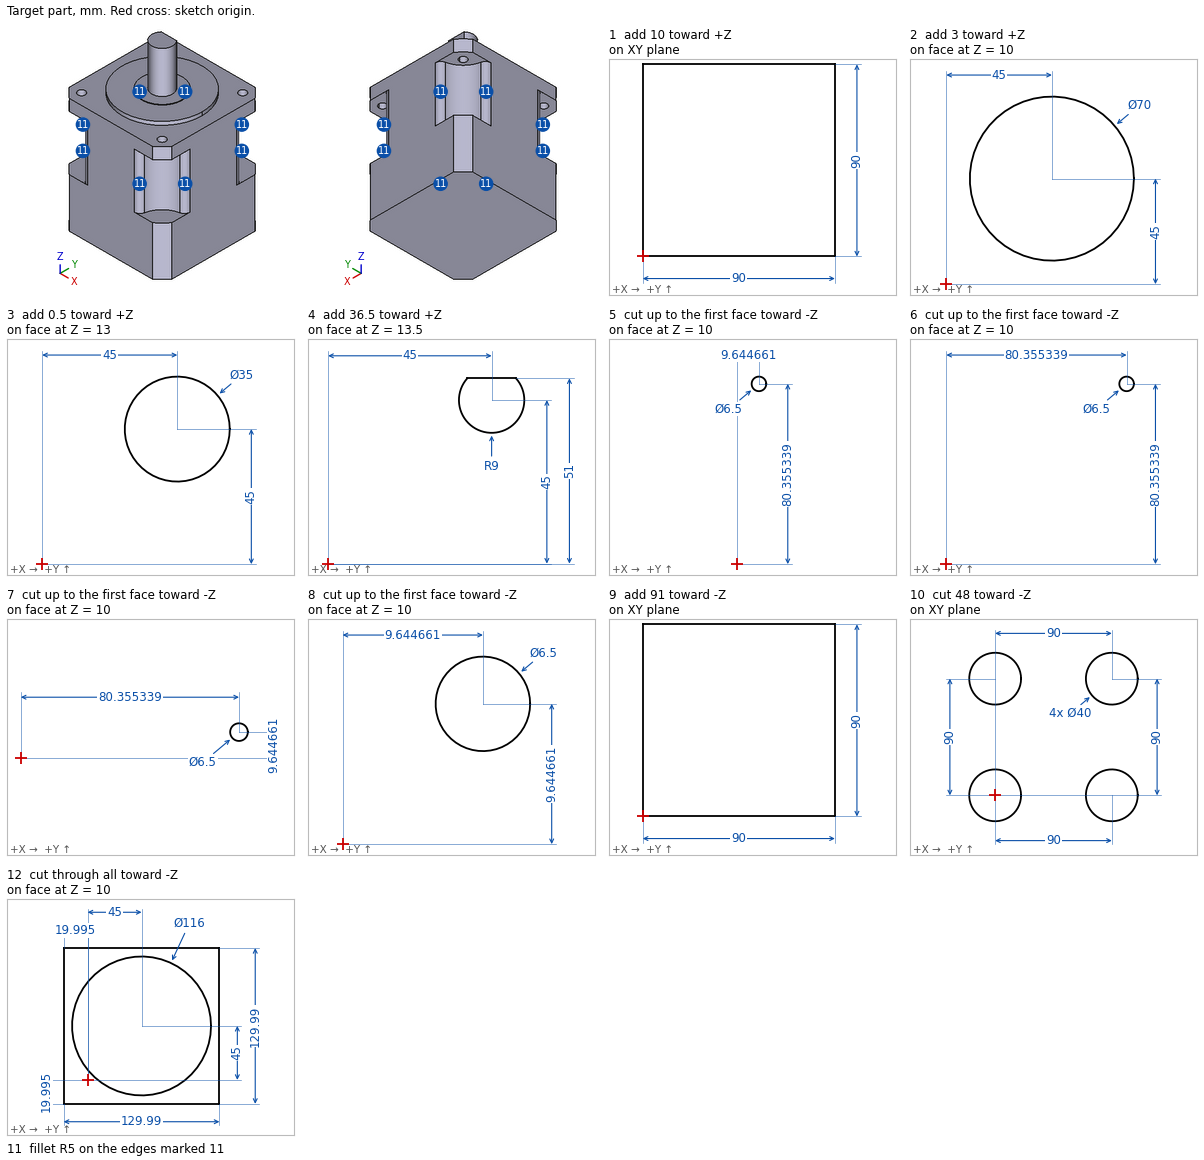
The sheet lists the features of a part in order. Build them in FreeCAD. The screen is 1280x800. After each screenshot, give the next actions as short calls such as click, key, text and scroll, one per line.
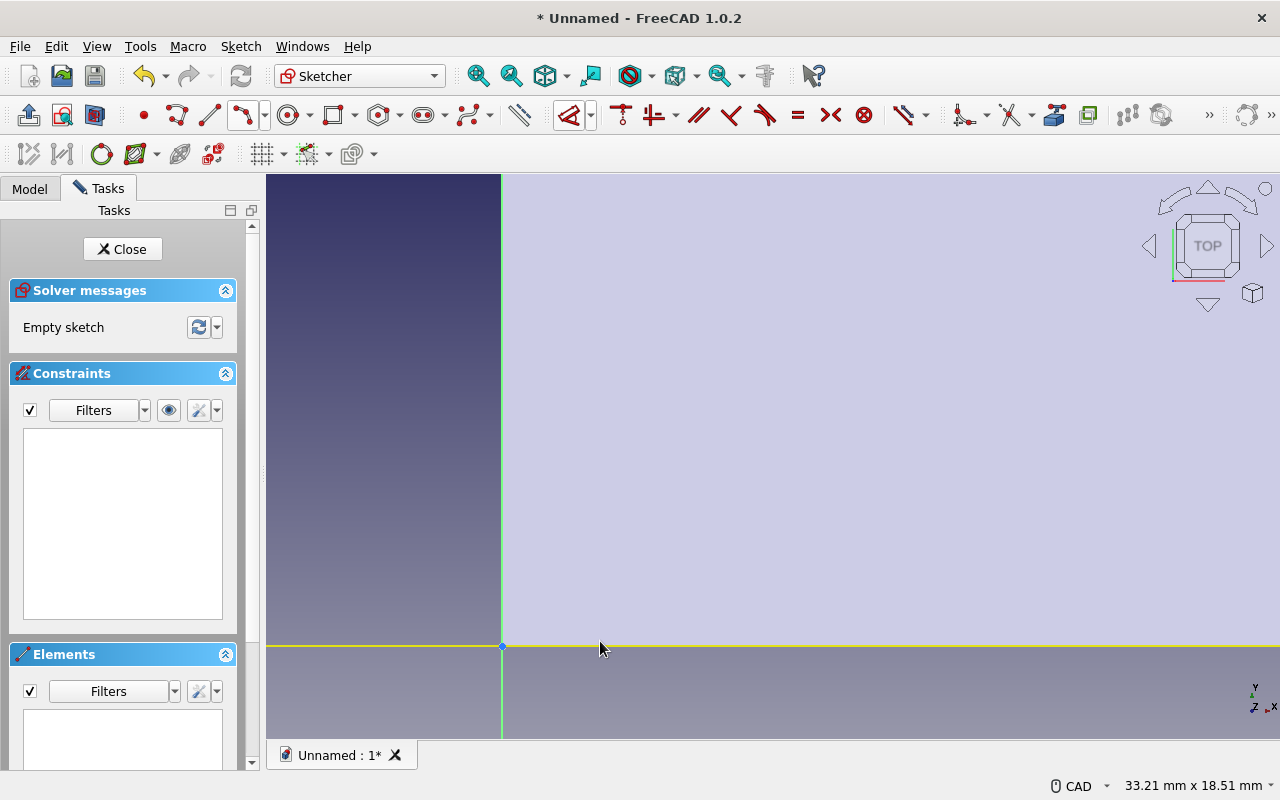
key(g)
key(c)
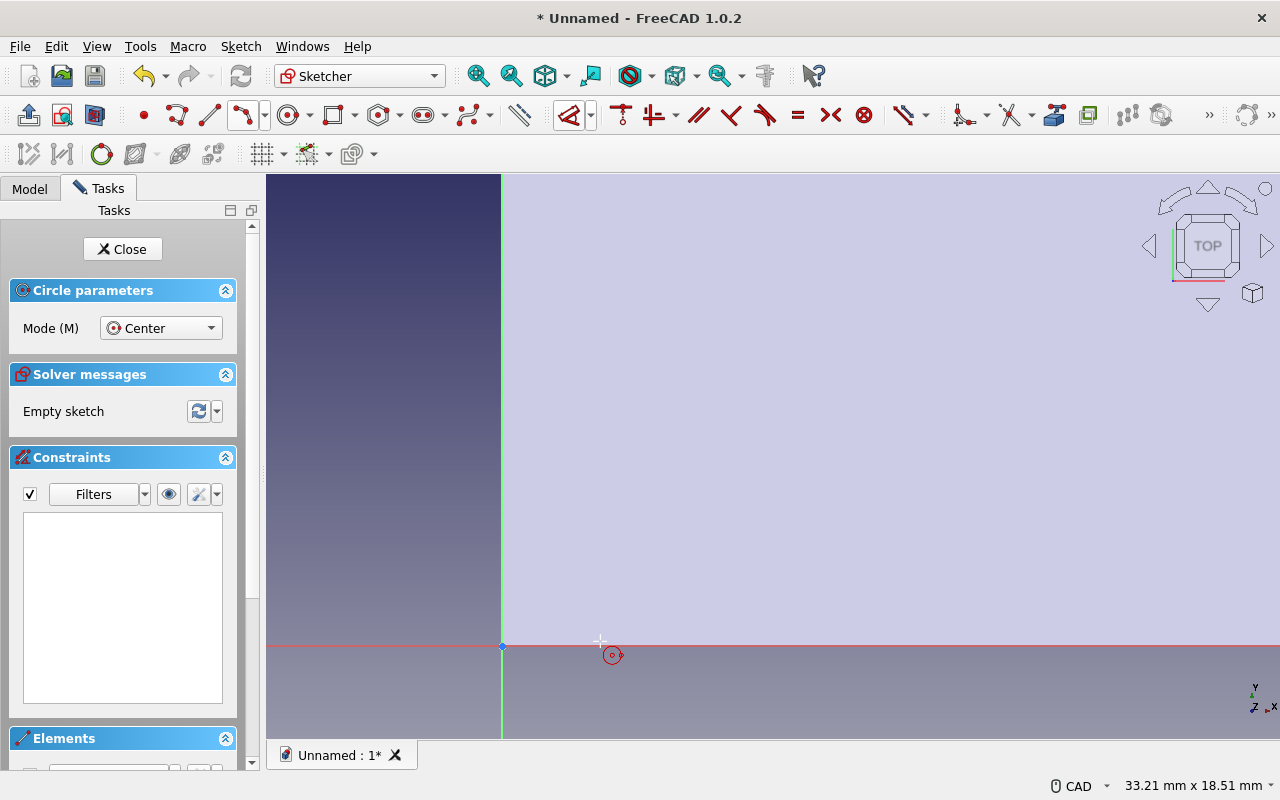
click(797, 352)
move(867, 282)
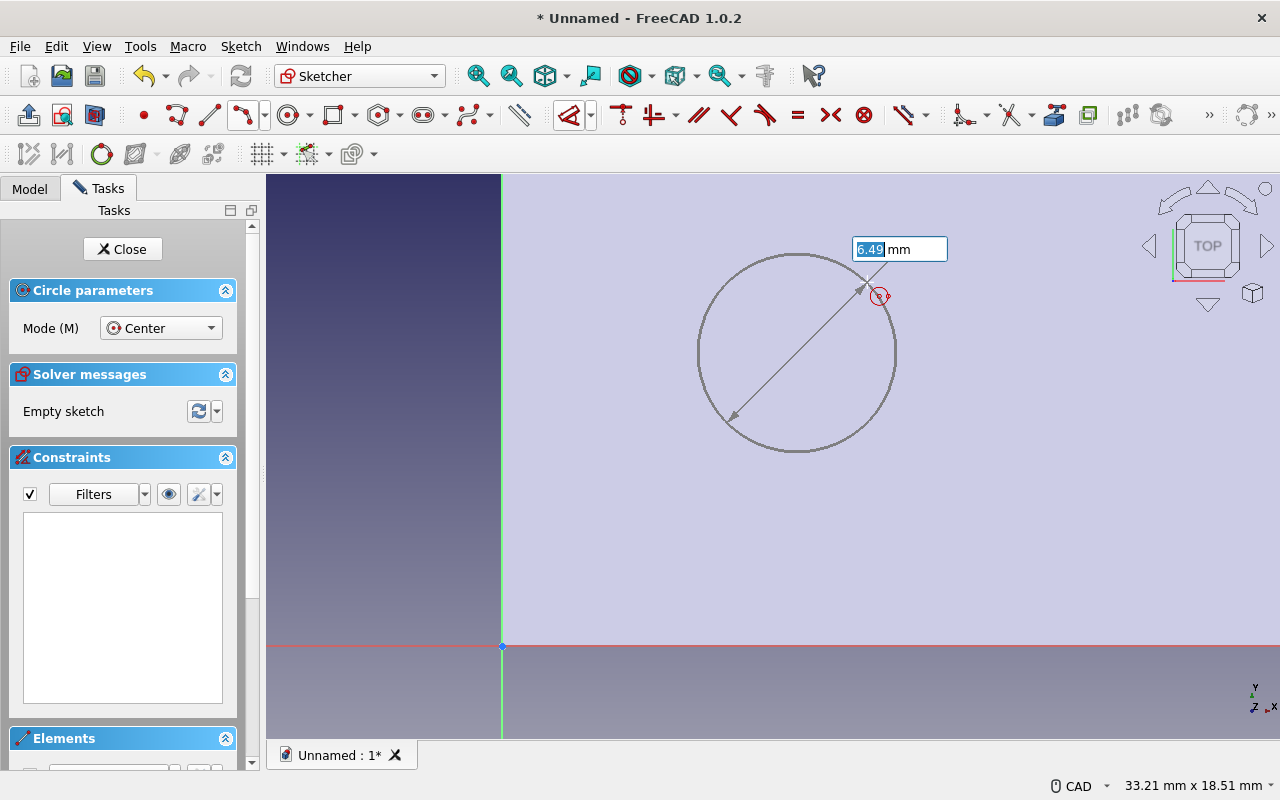
text(6.5)
key(Return)
key(Escape)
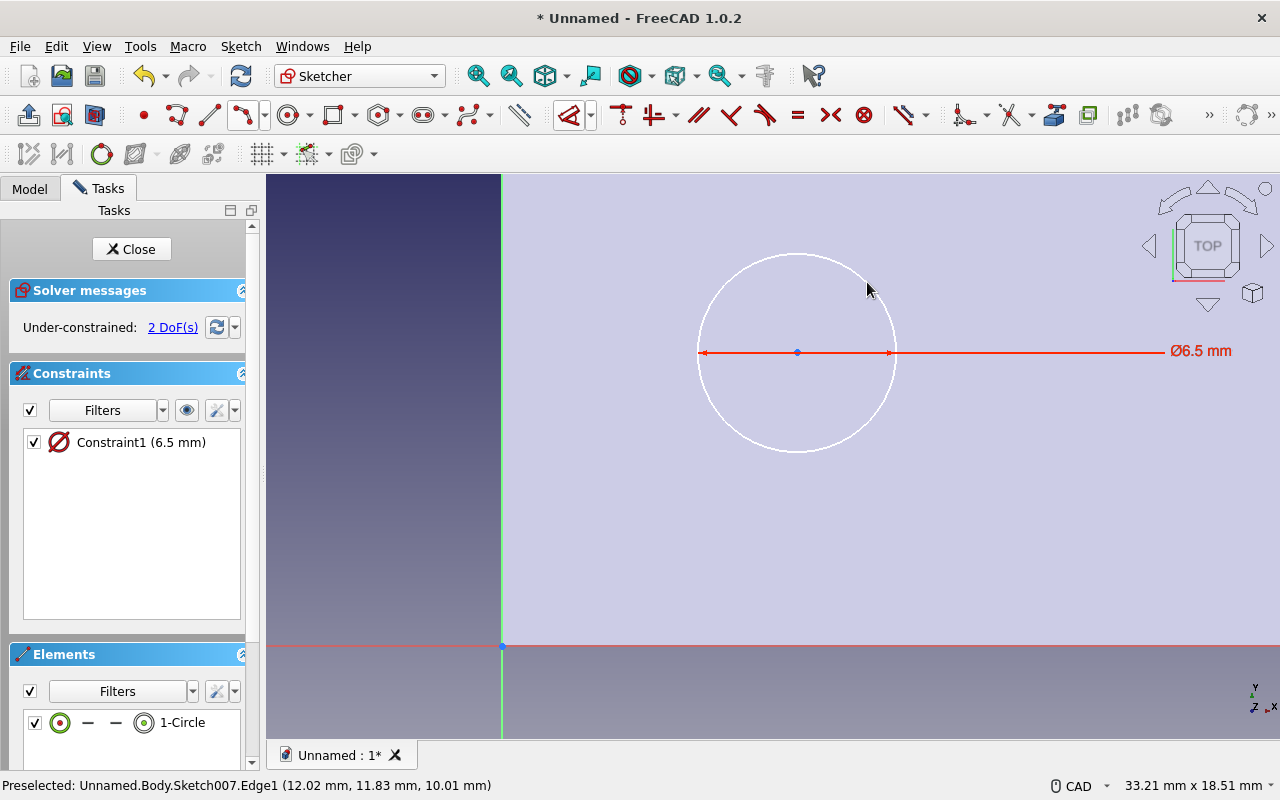
click(797, 353)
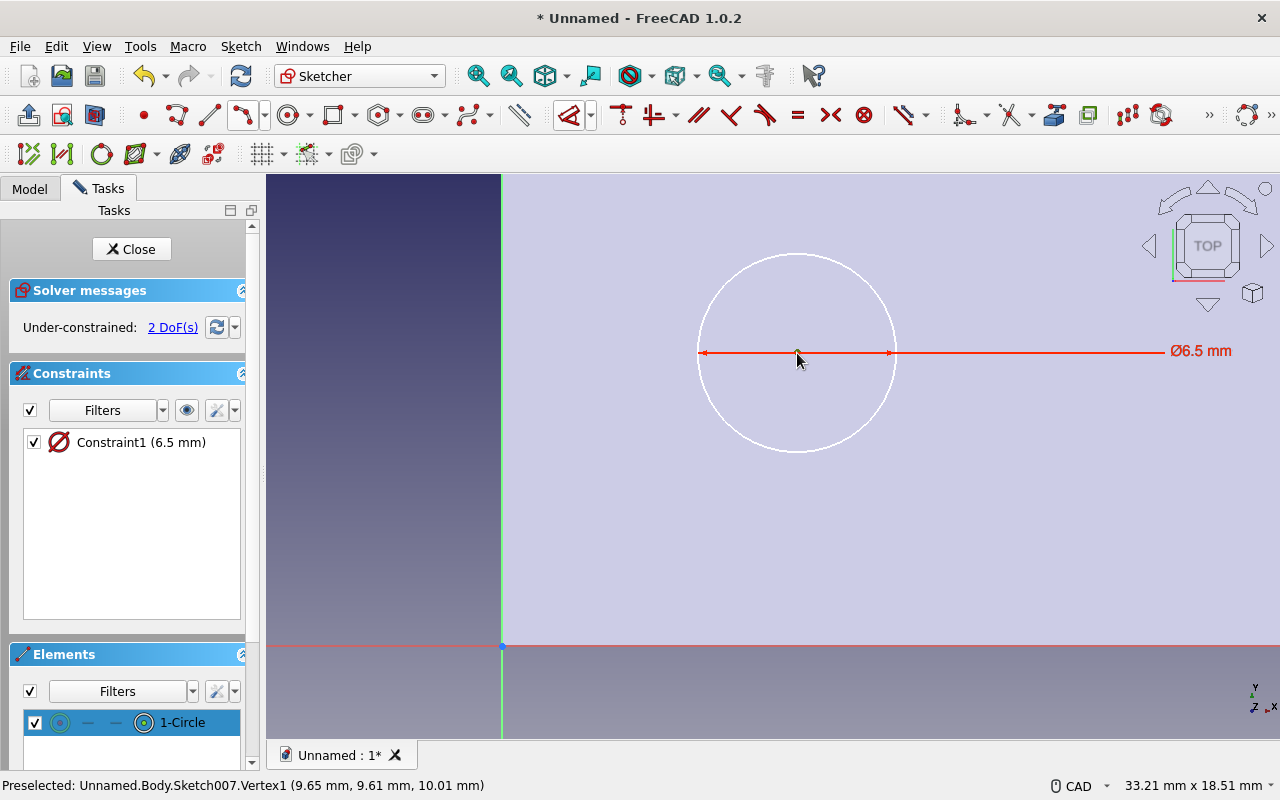
key(l)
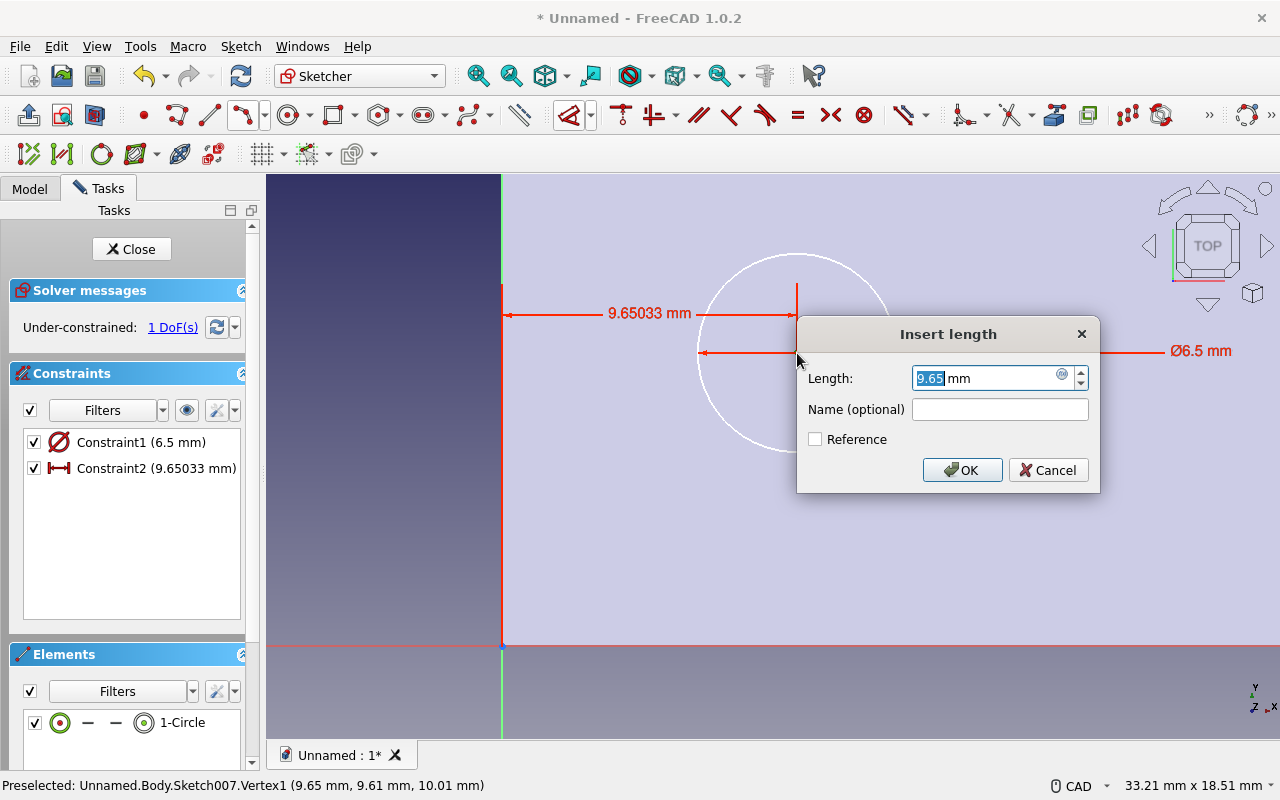
text(9.644661)
key(Return)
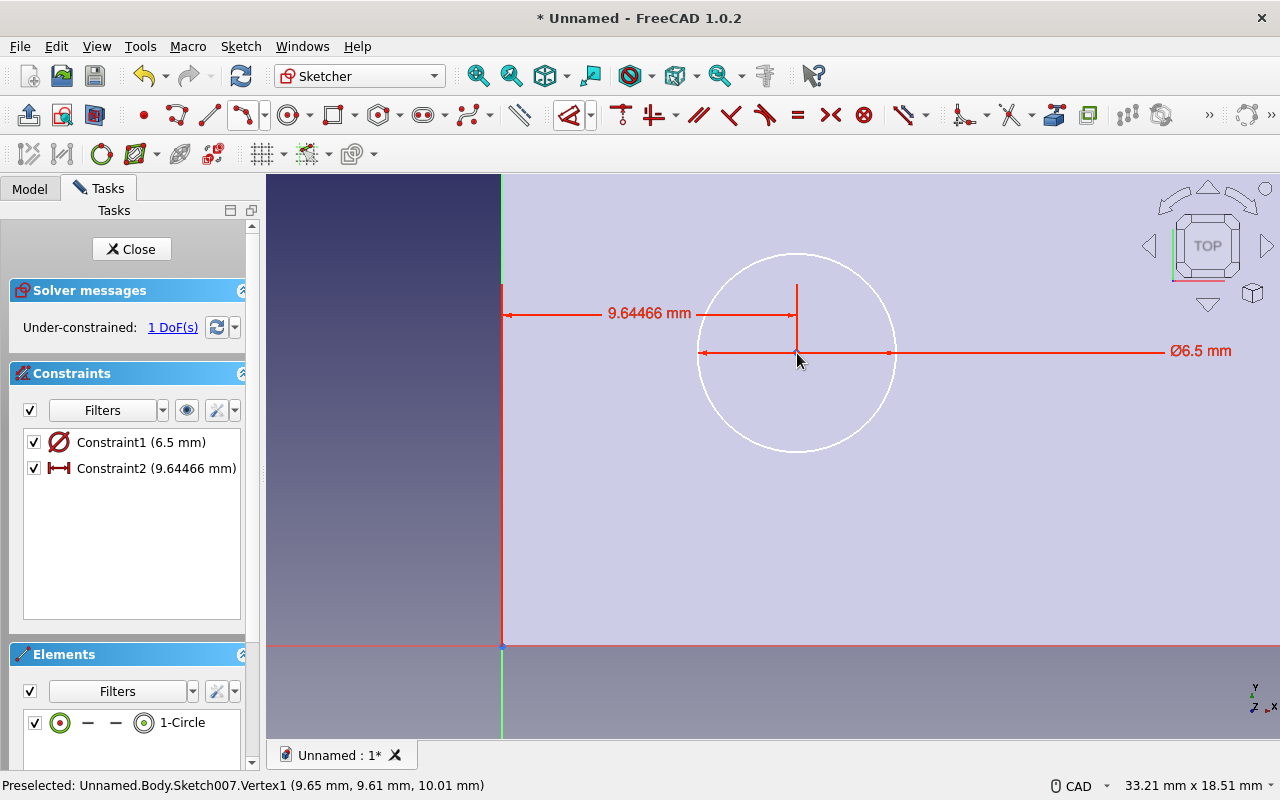
click(797, 353)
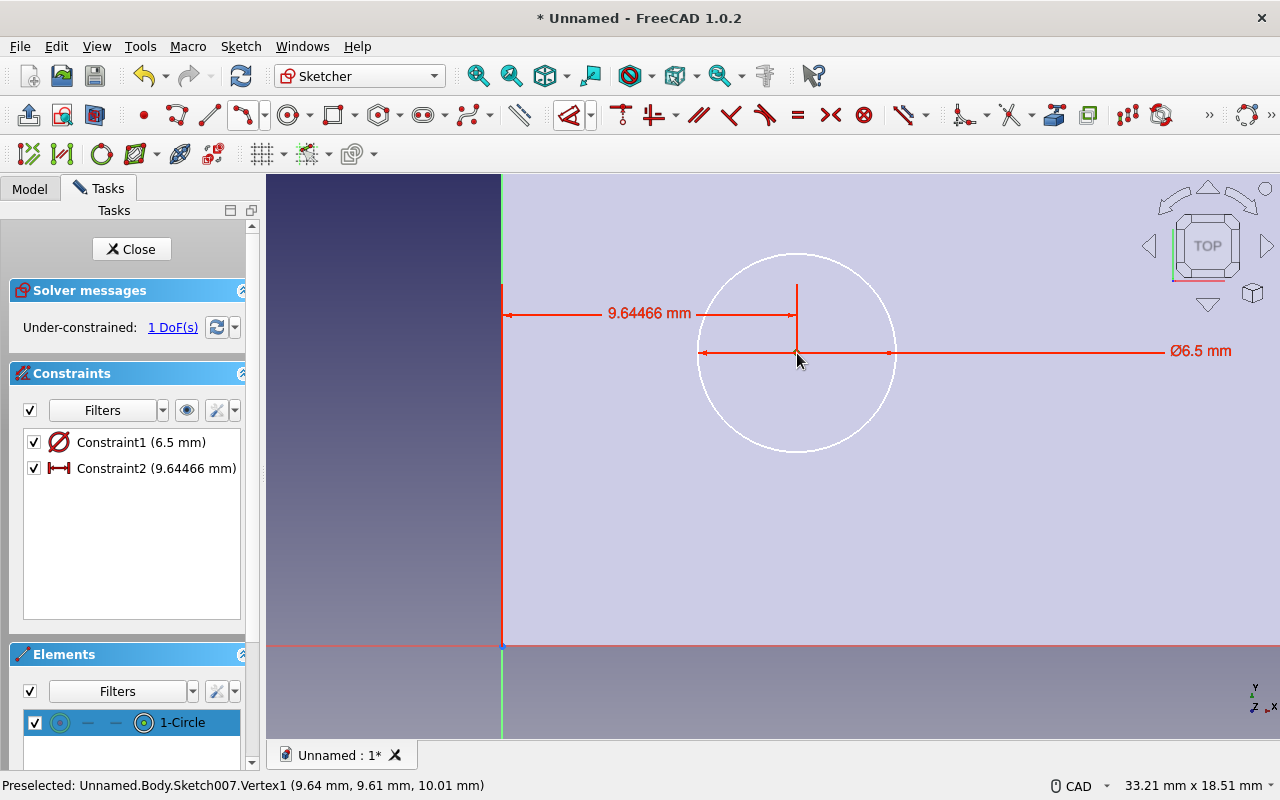
key(i)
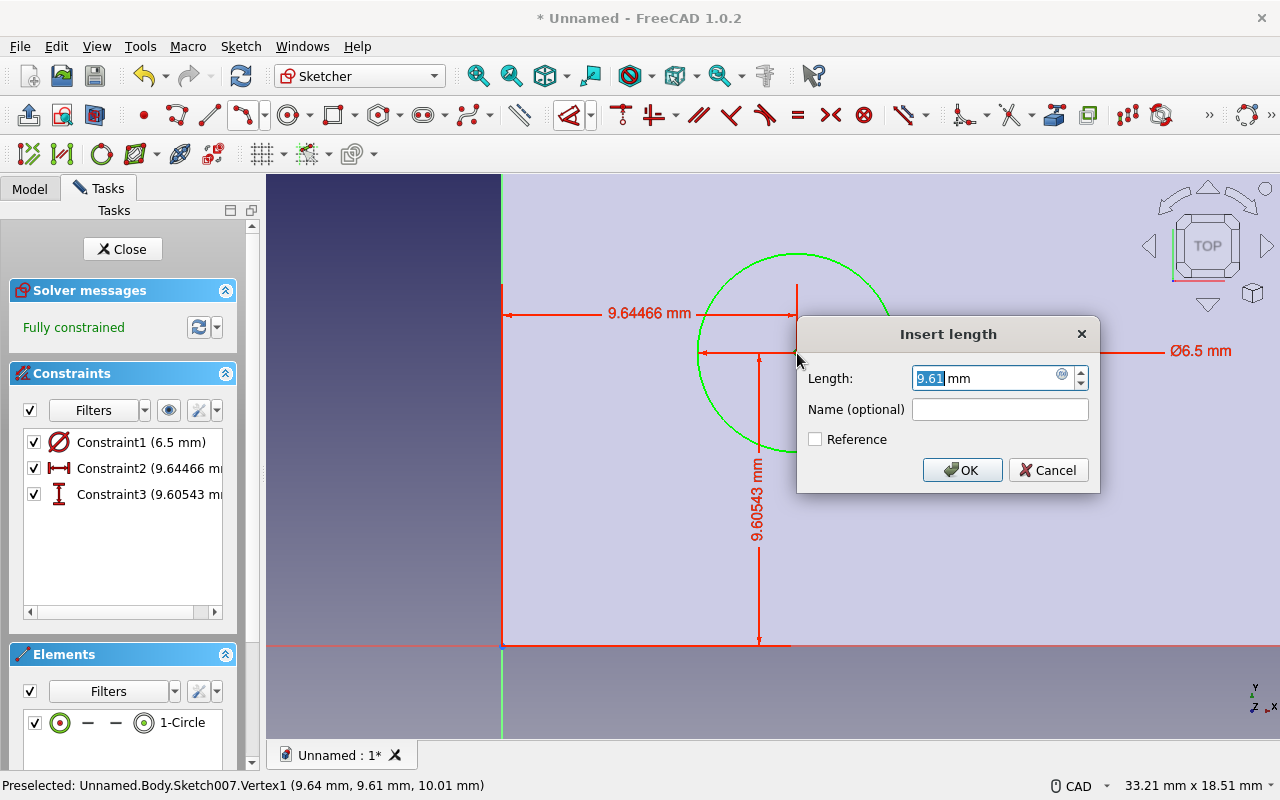
text(9.644661)
key(Return)